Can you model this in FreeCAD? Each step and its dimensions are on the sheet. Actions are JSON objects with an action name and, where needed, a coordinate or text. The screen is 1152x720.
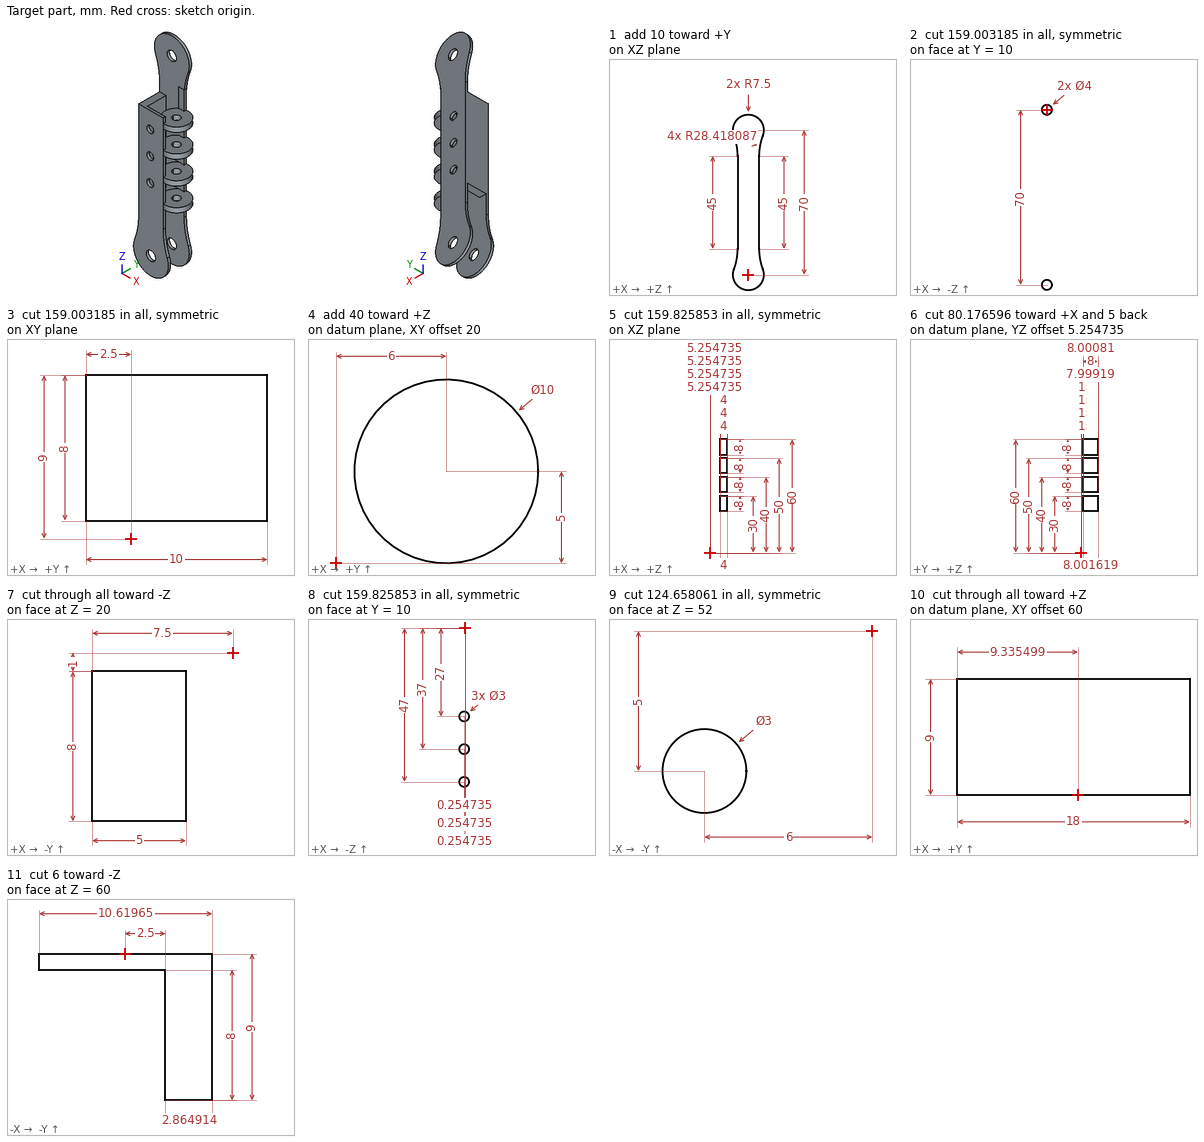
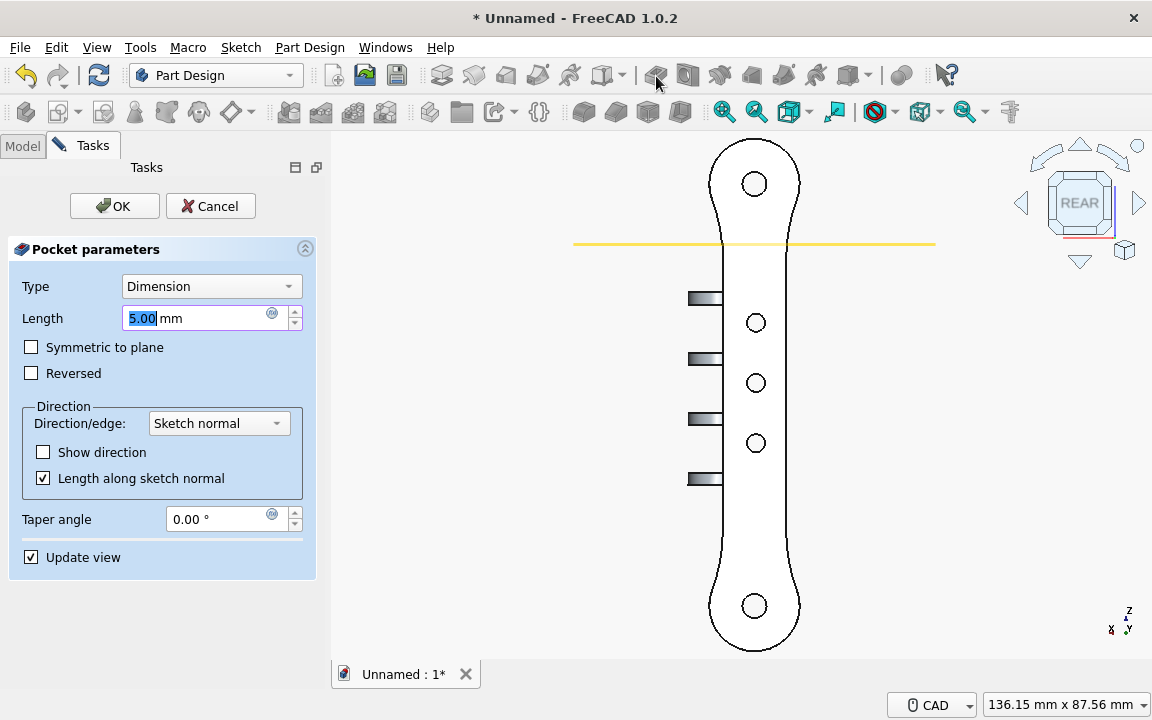
{"action": "left_click", "coordinate": [212, 286]}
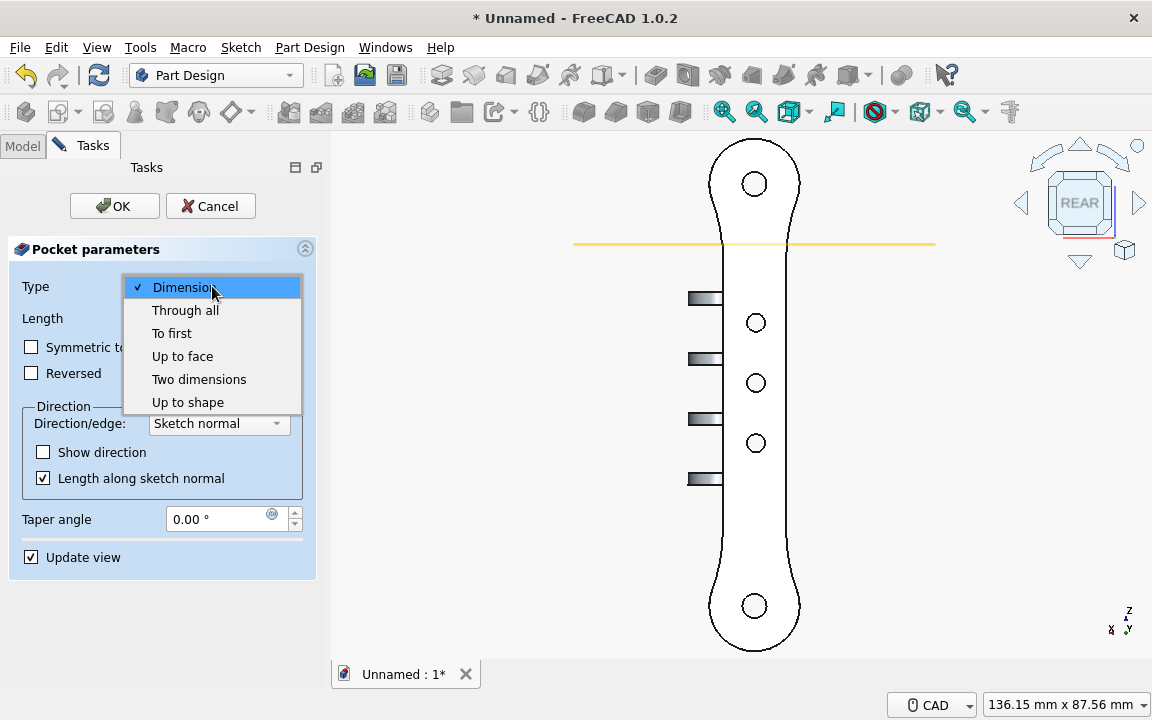
{"action": "left_click", "coordinate": [212, 310]}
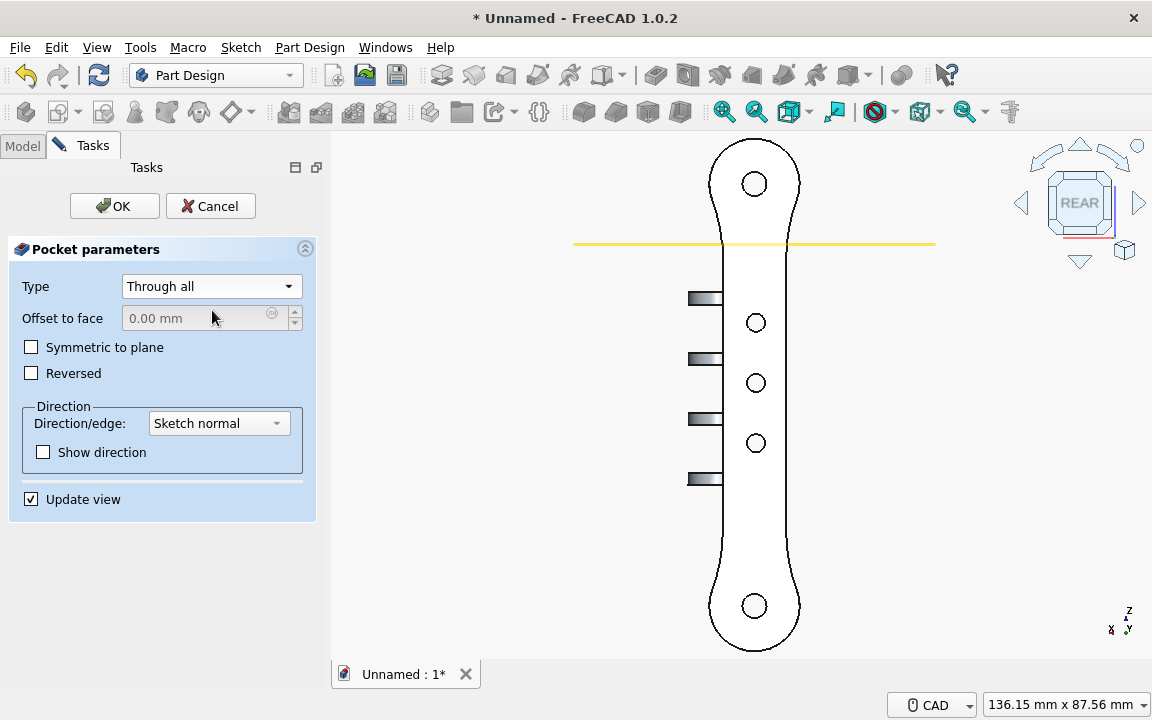
{"action": "left_click", "coordinate": [30, 373]}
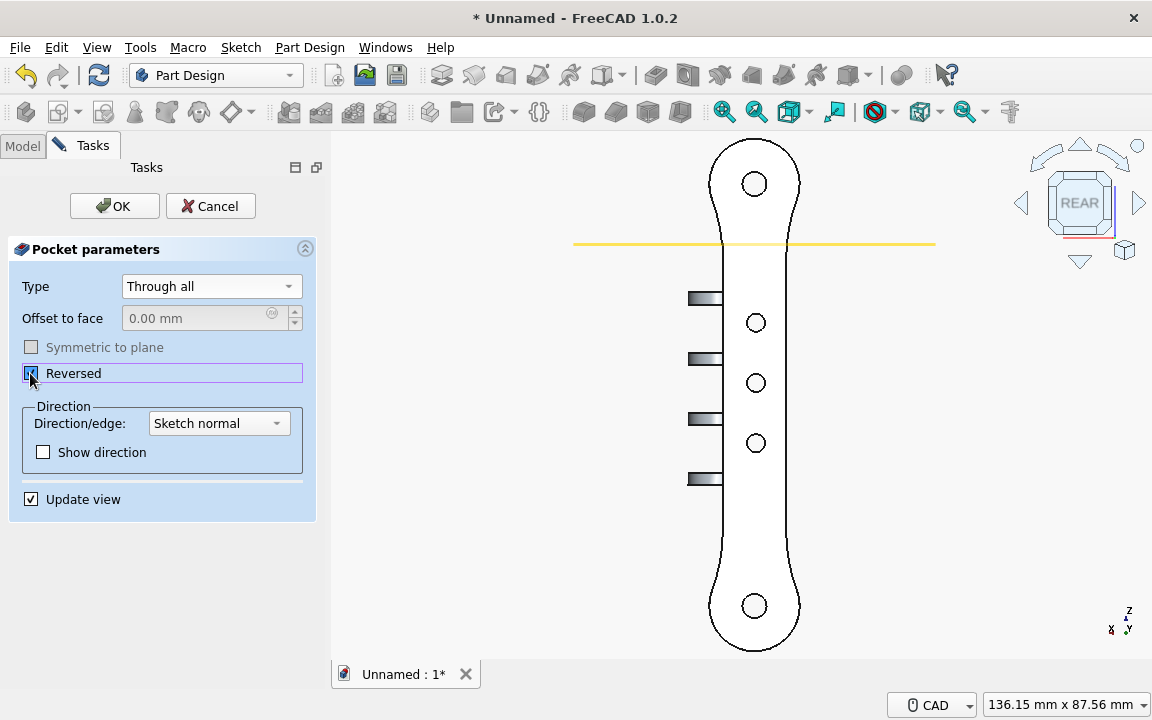
{"action": "left_click", "coordinate": [115, 206]}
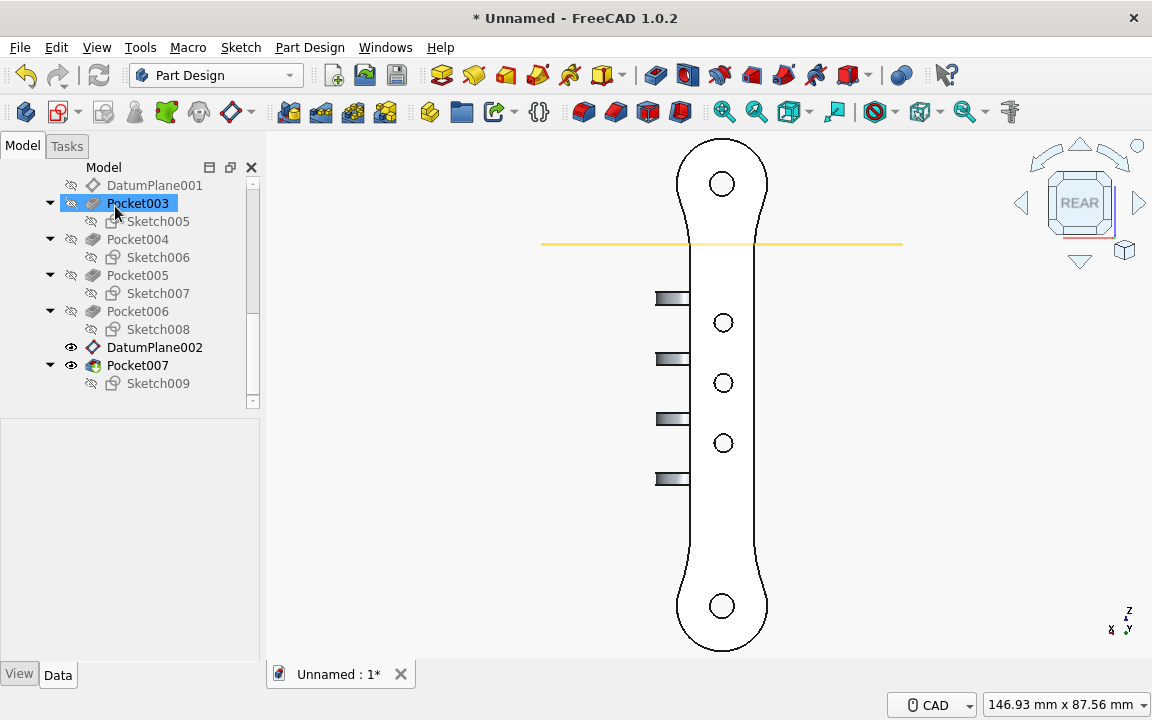
{"action": "left_click", "coordinate": [116, 347]}
{"action": "key", "text": "space"}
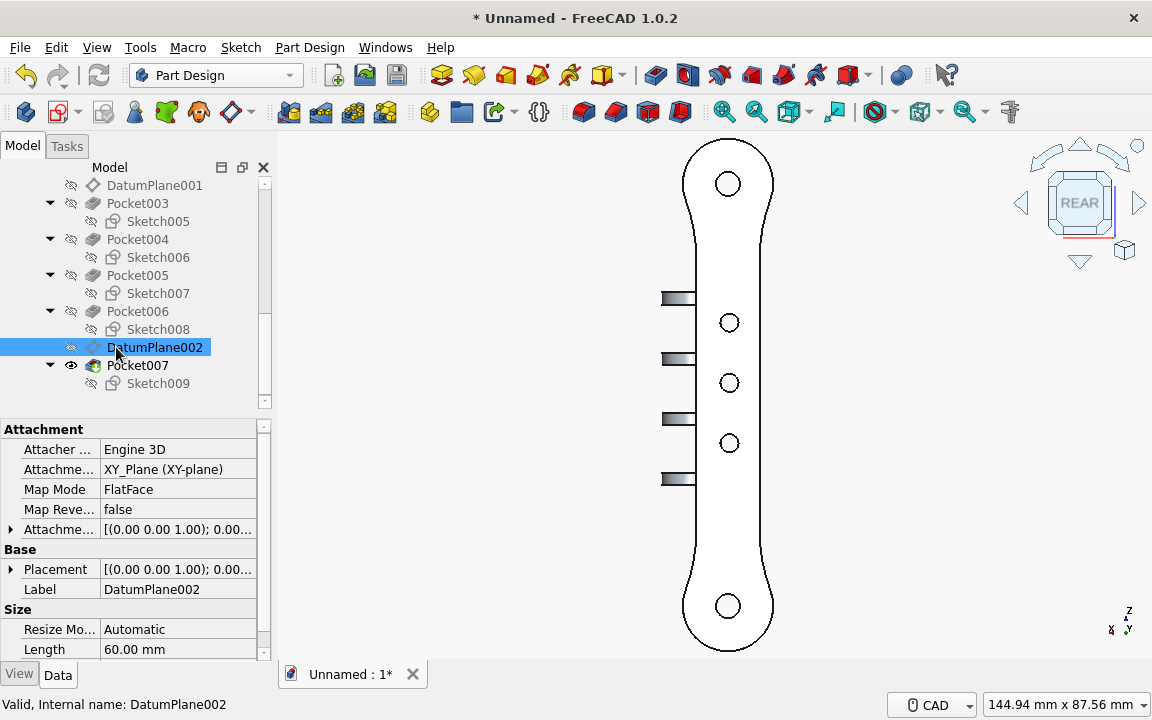
{"action": "key", "text": "0"}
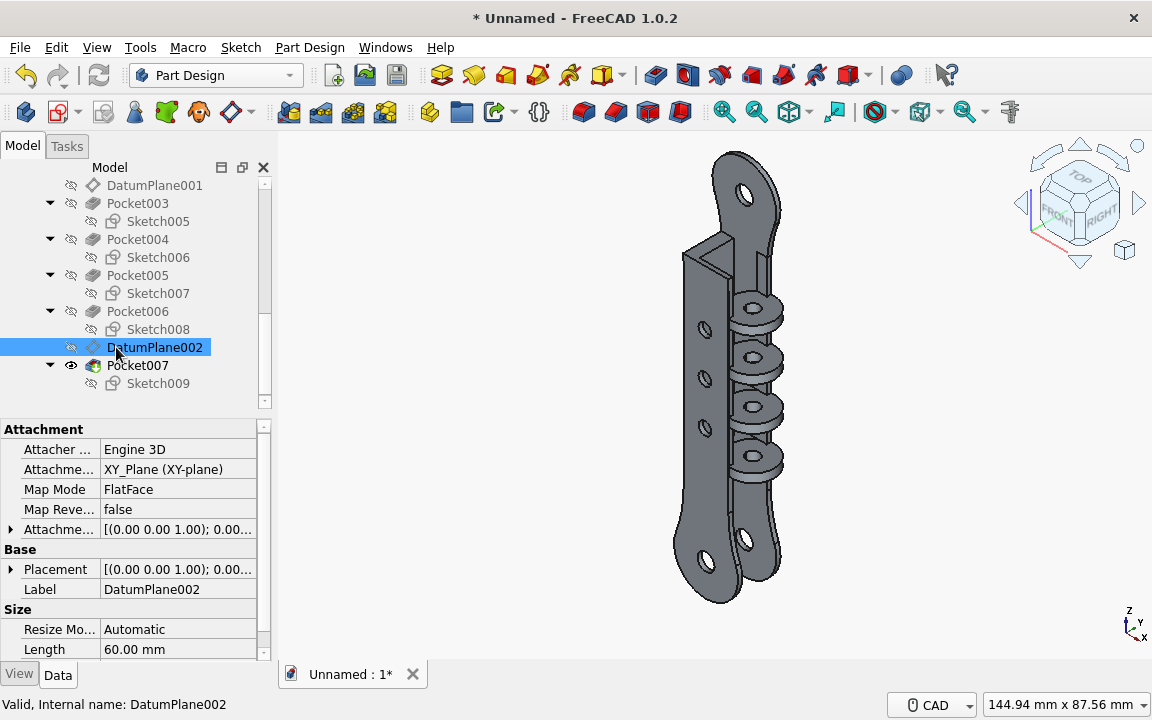
{"action": "scroll", "coordinate": [716, 237], "scroll_direction": "up", "scroll_amount": 5}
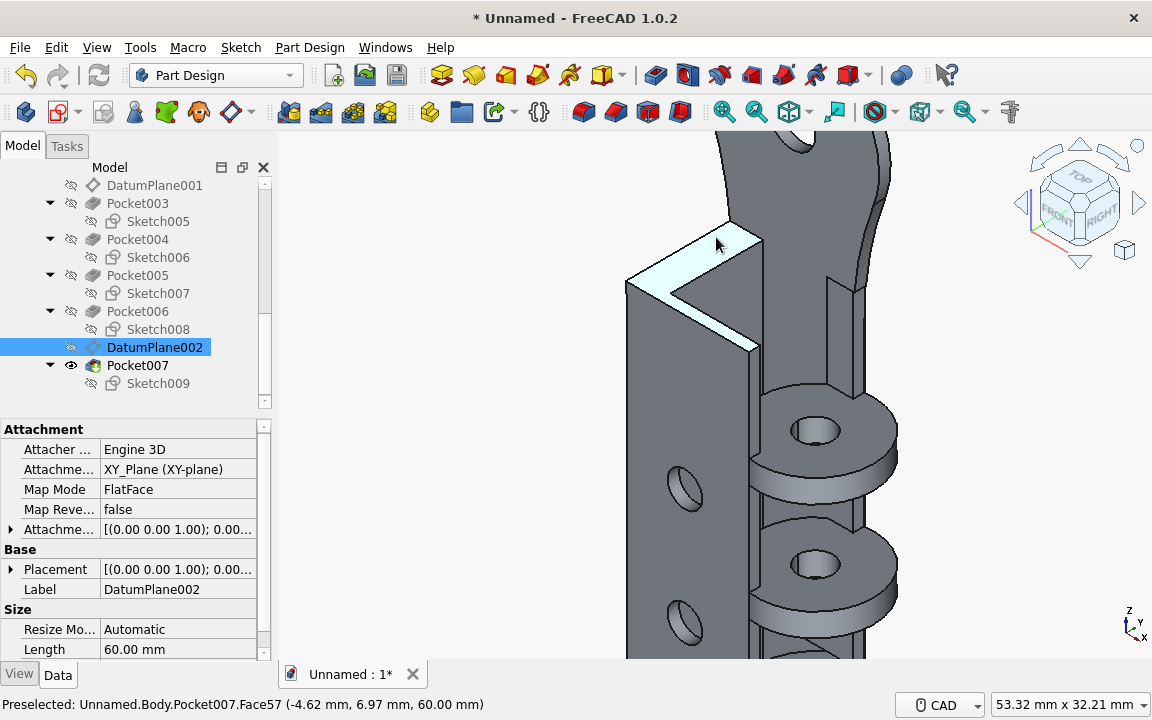
{"action": "left_click", "coordinate": [716, 238]}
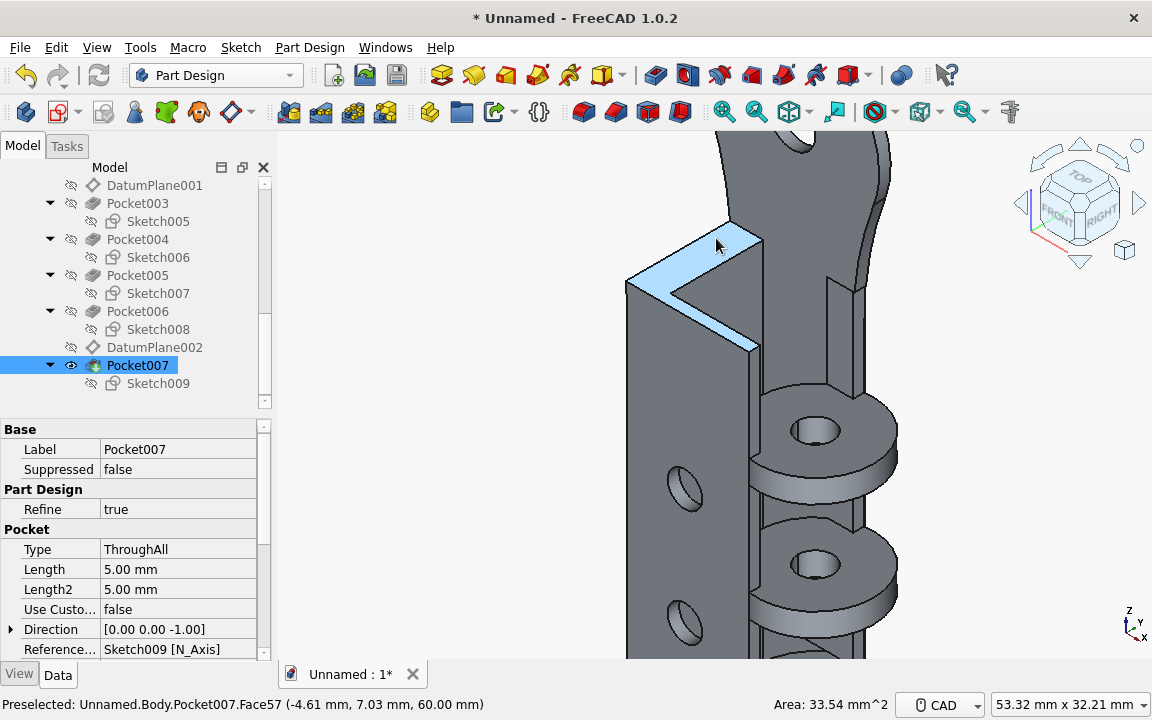
{"action": "left_click", "coordinate": [58, 112]}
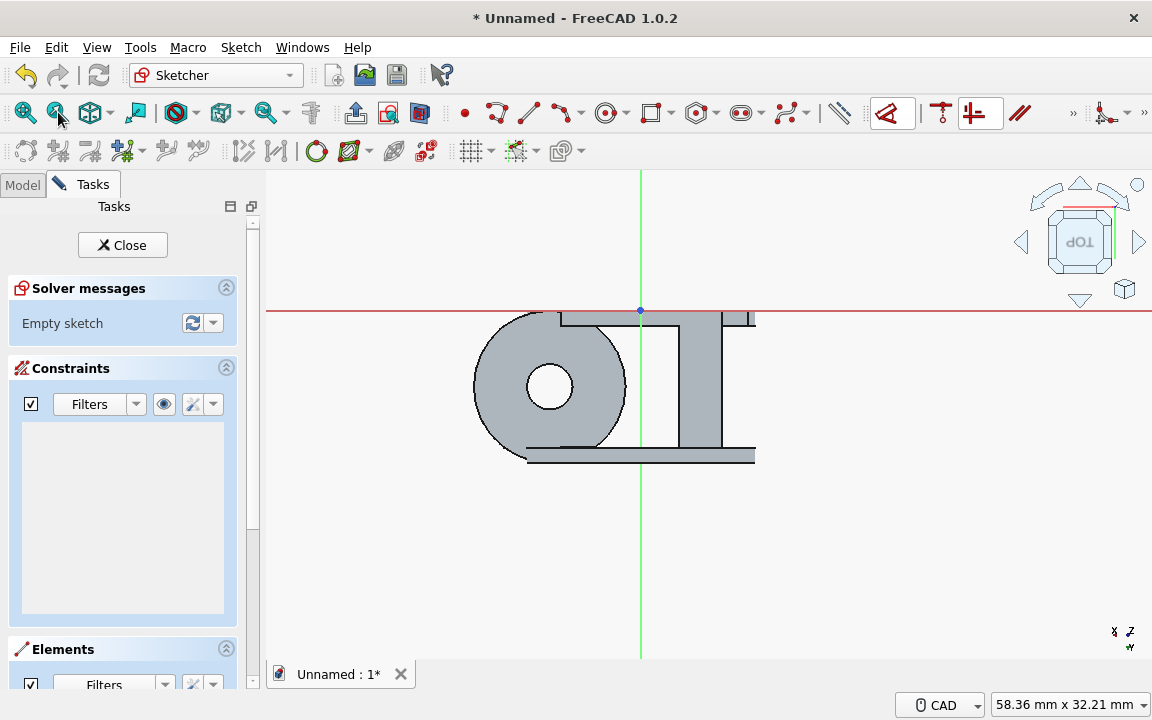
{"action": "scroll", "coordinate": [643, 350], "scroll_direction": "up", "scroll_amount": 4}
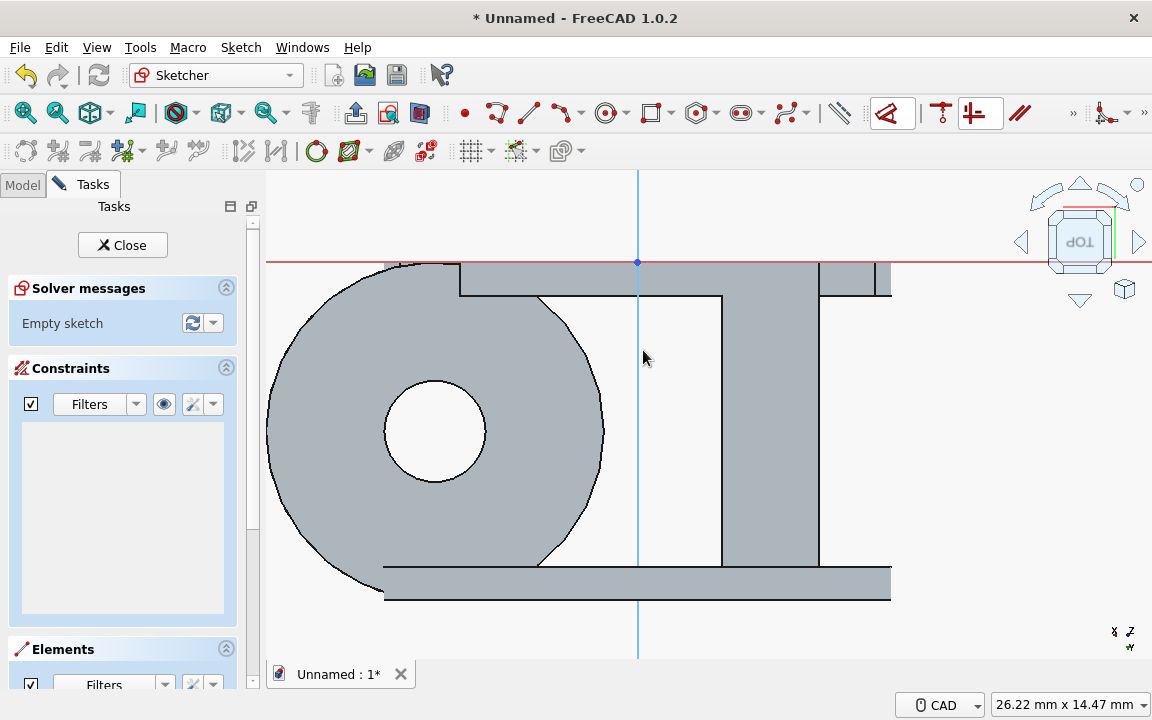
{"action": "left_click", "coordinate": [498, 114]}